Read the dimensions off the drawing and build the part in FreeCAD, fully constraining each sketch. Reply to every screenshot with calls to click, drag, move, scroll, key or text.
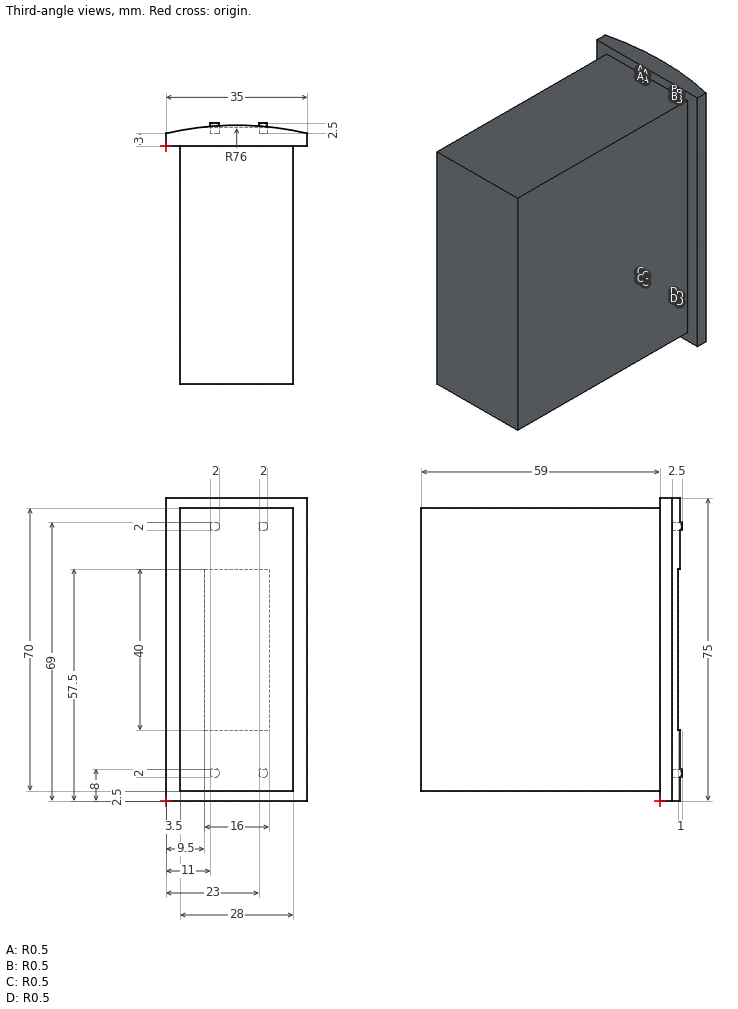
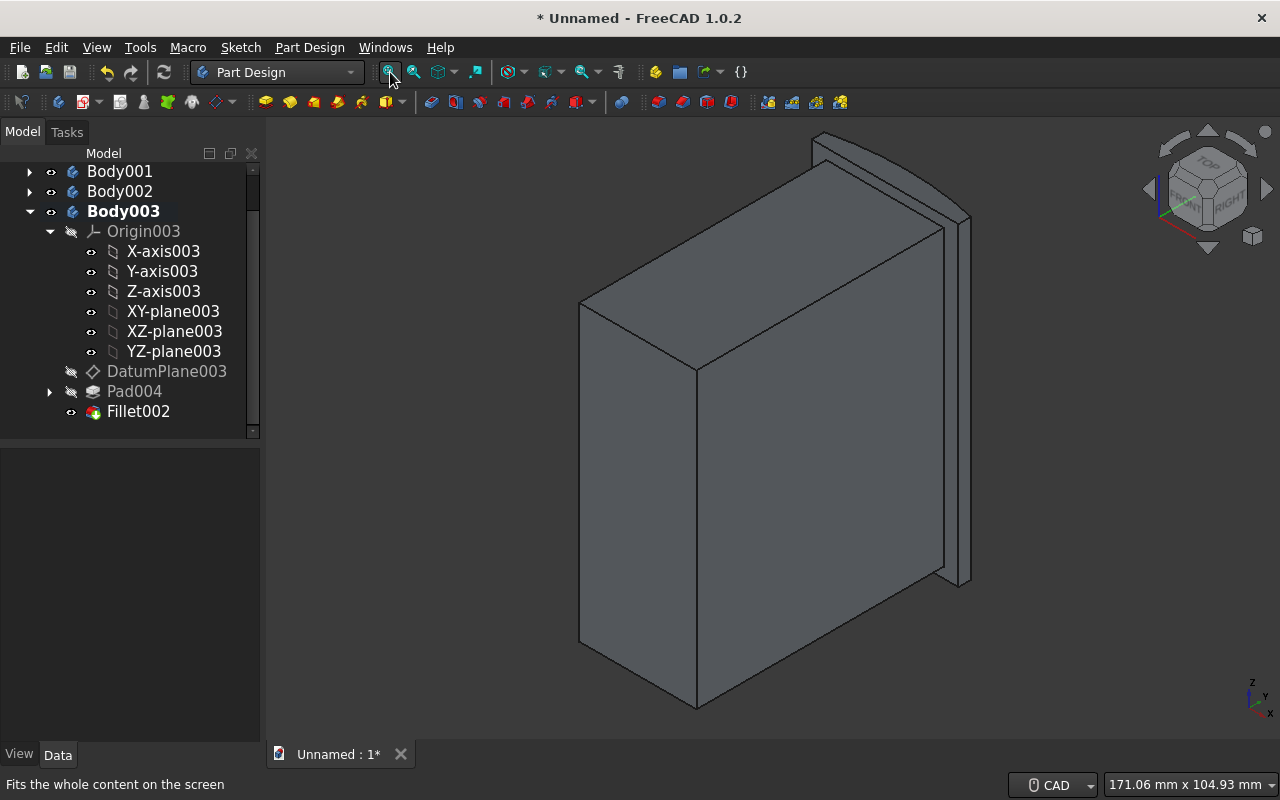
click(60, 102)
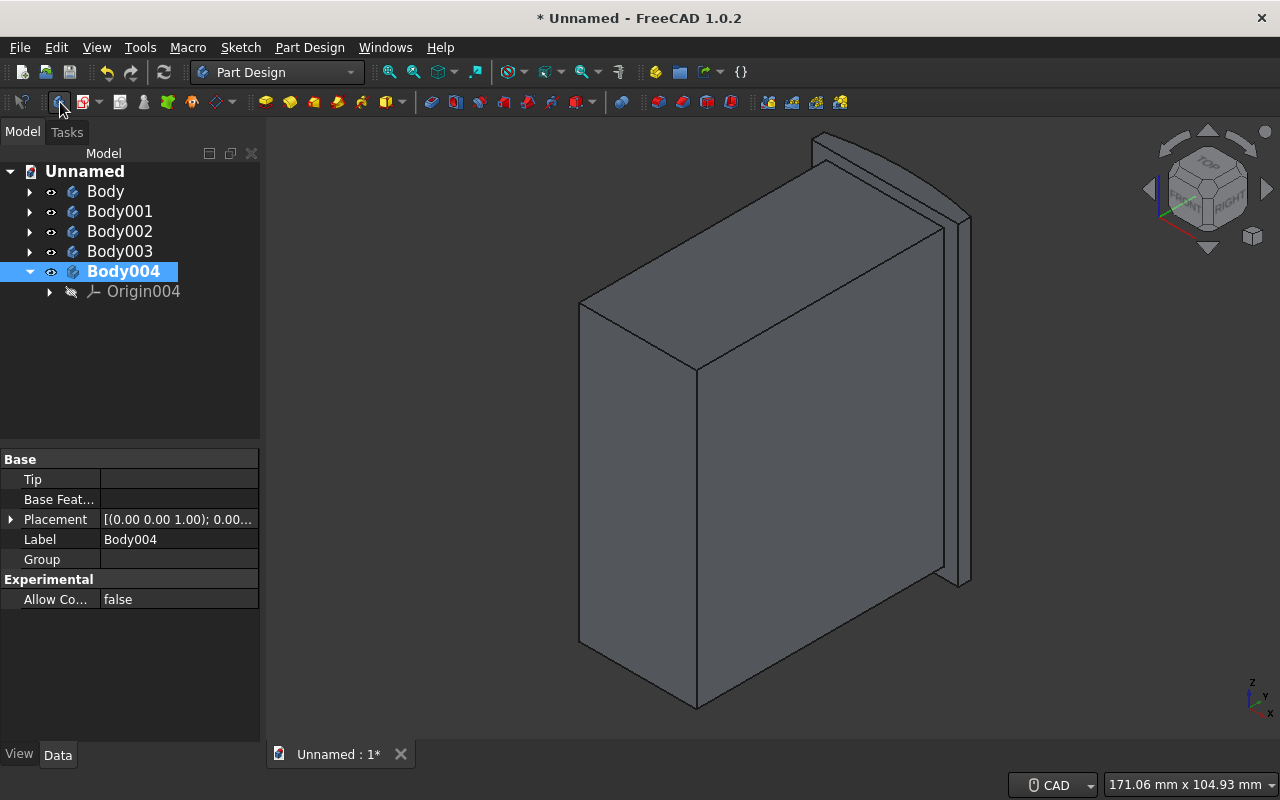
click(50, 292)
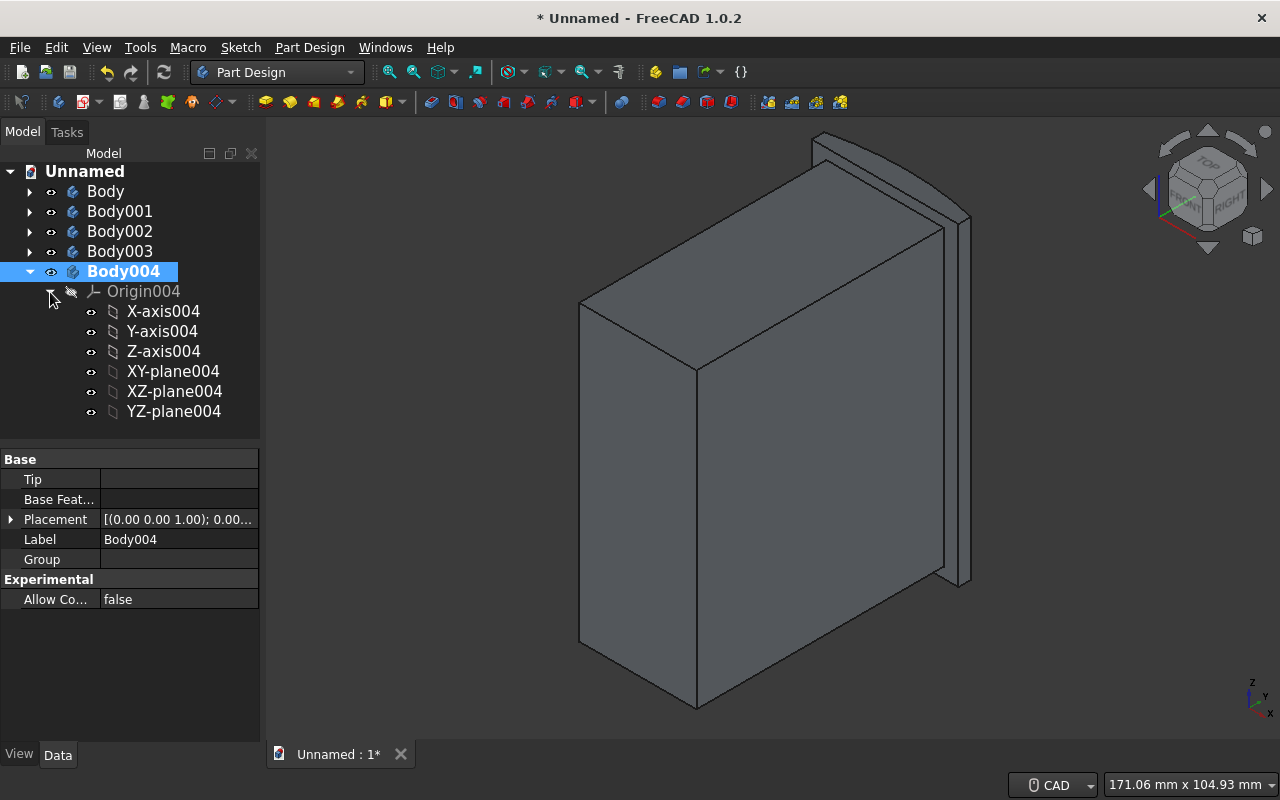
click(136, 392)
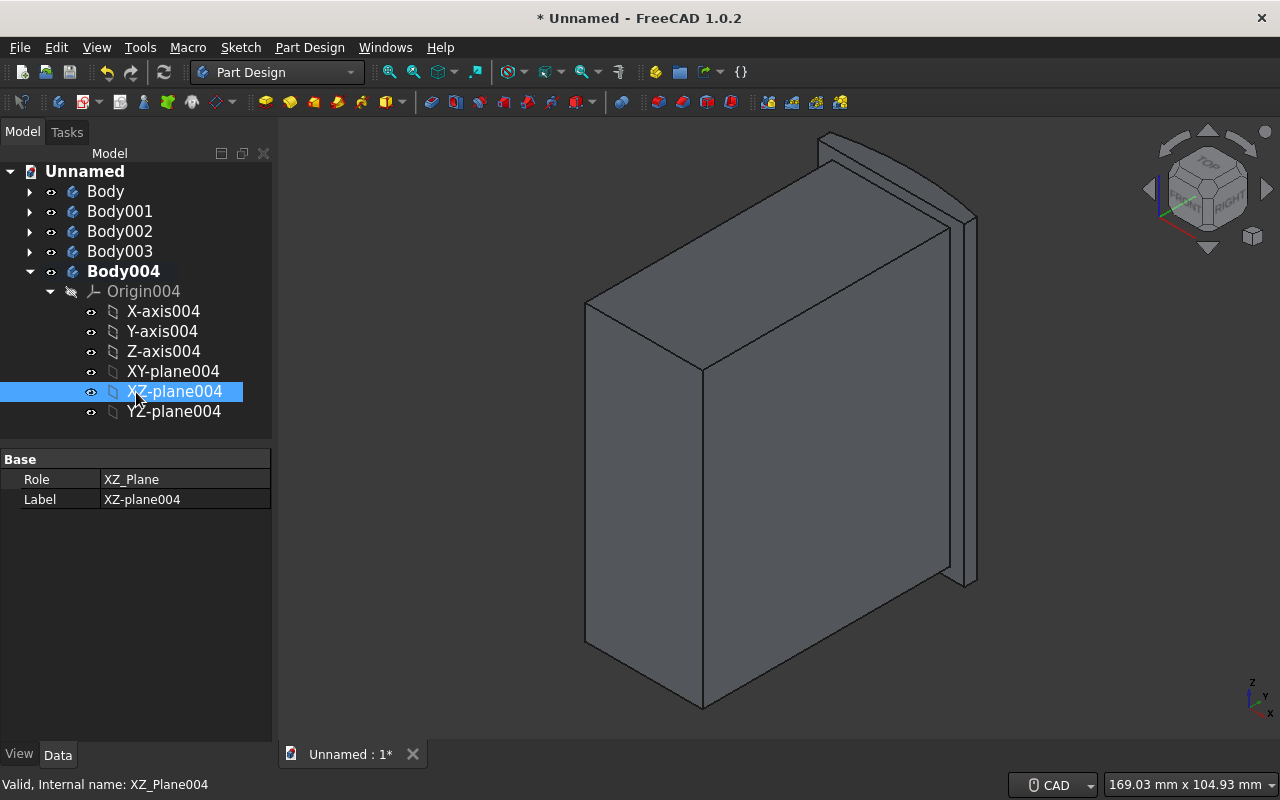
click(216, 102)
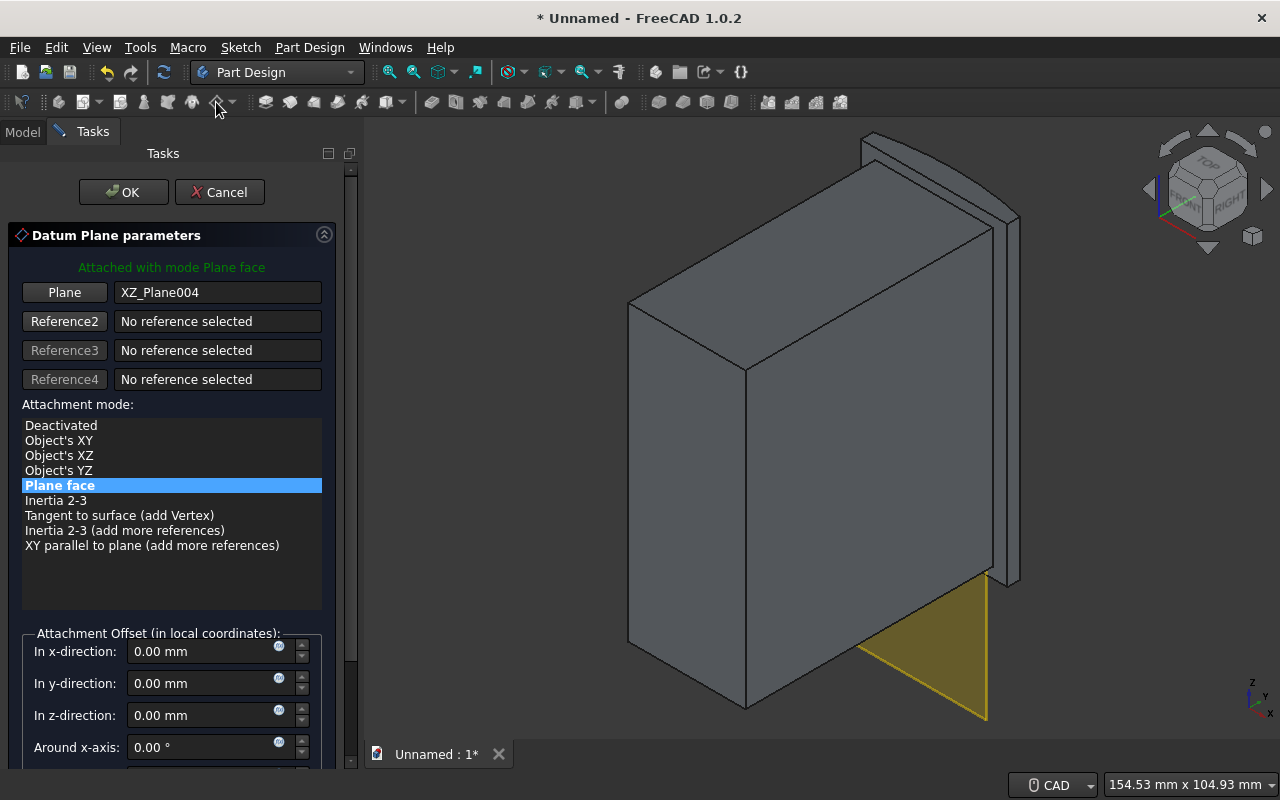
triple_click(210, 715)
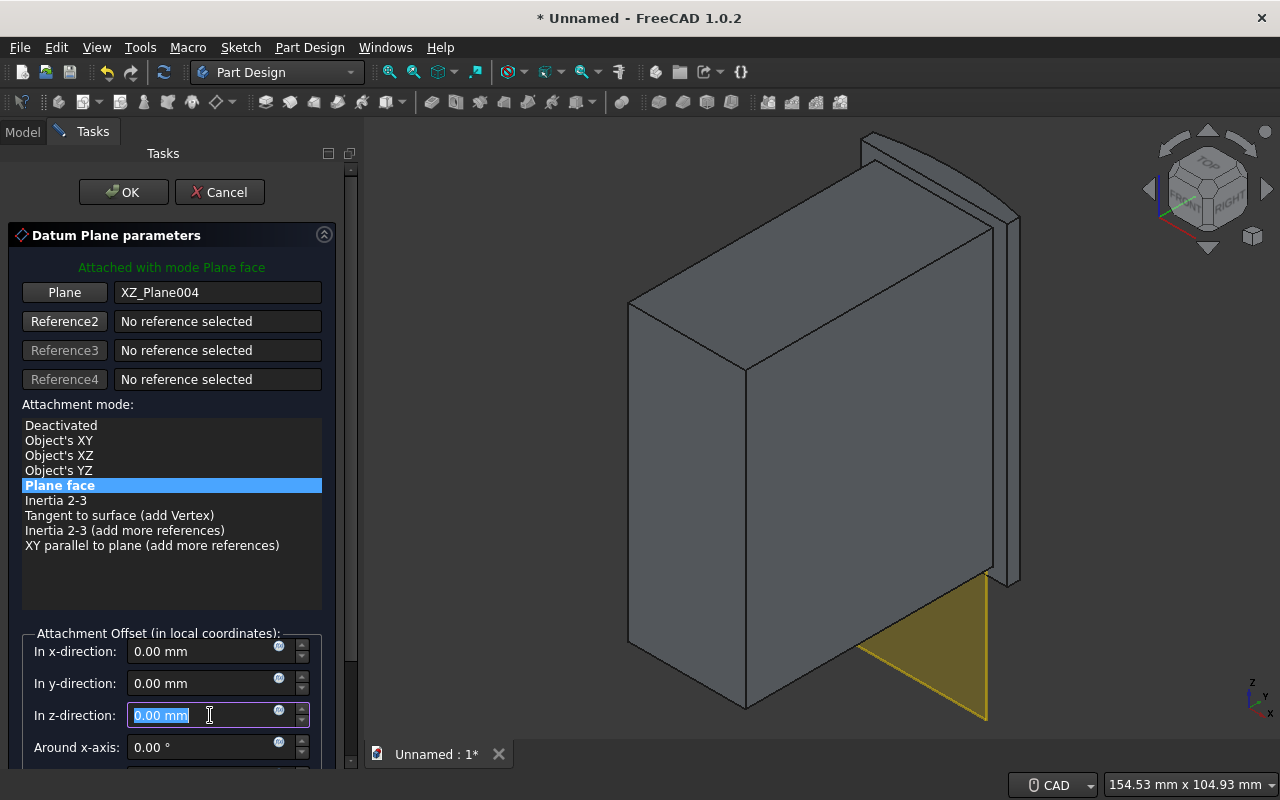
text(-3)
key(Tab)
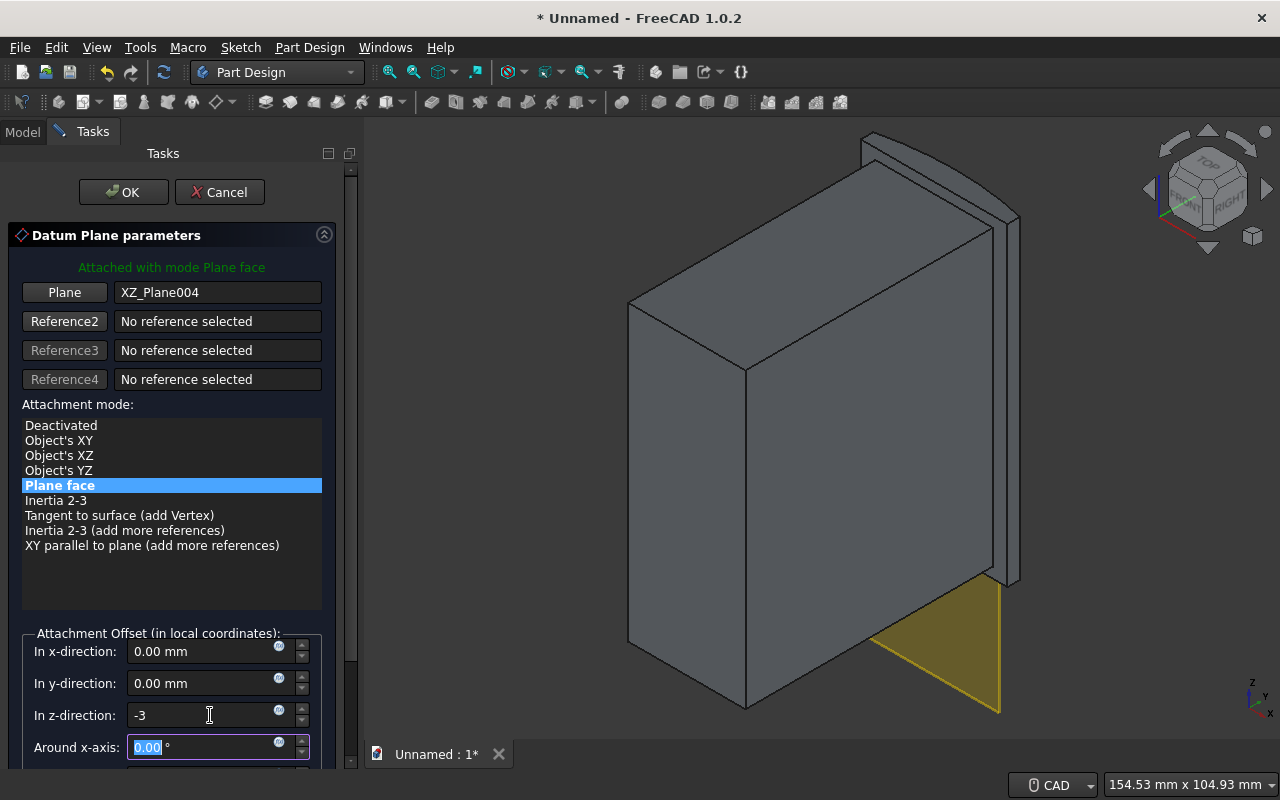
click(124, 192)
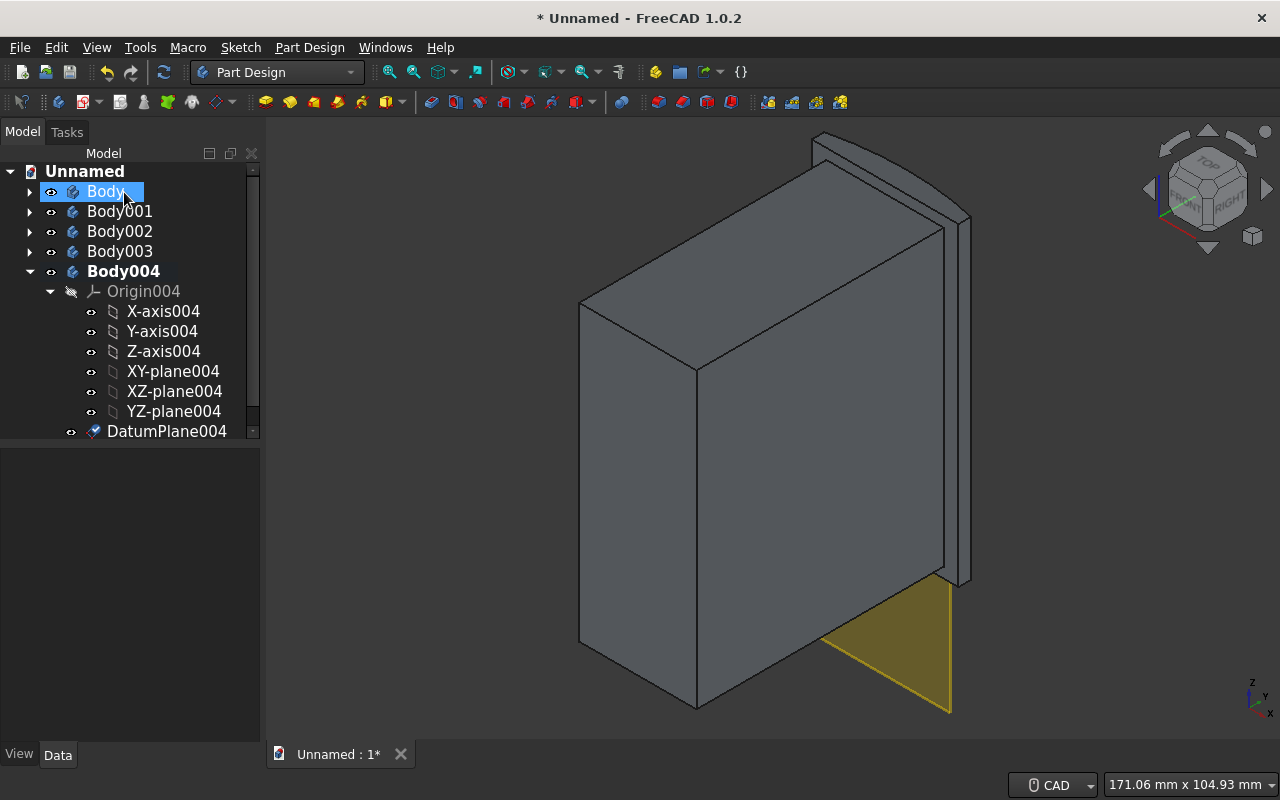
click(116, 432)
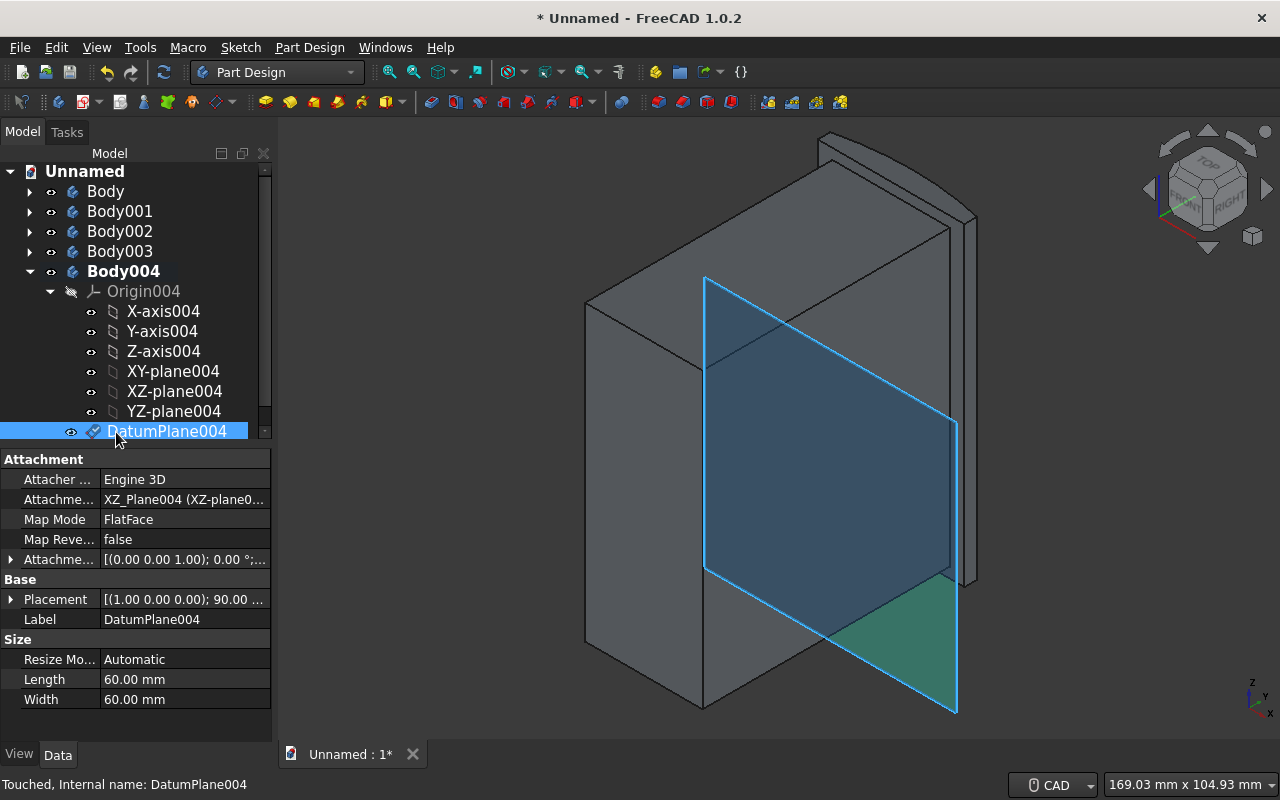
click(84, 102)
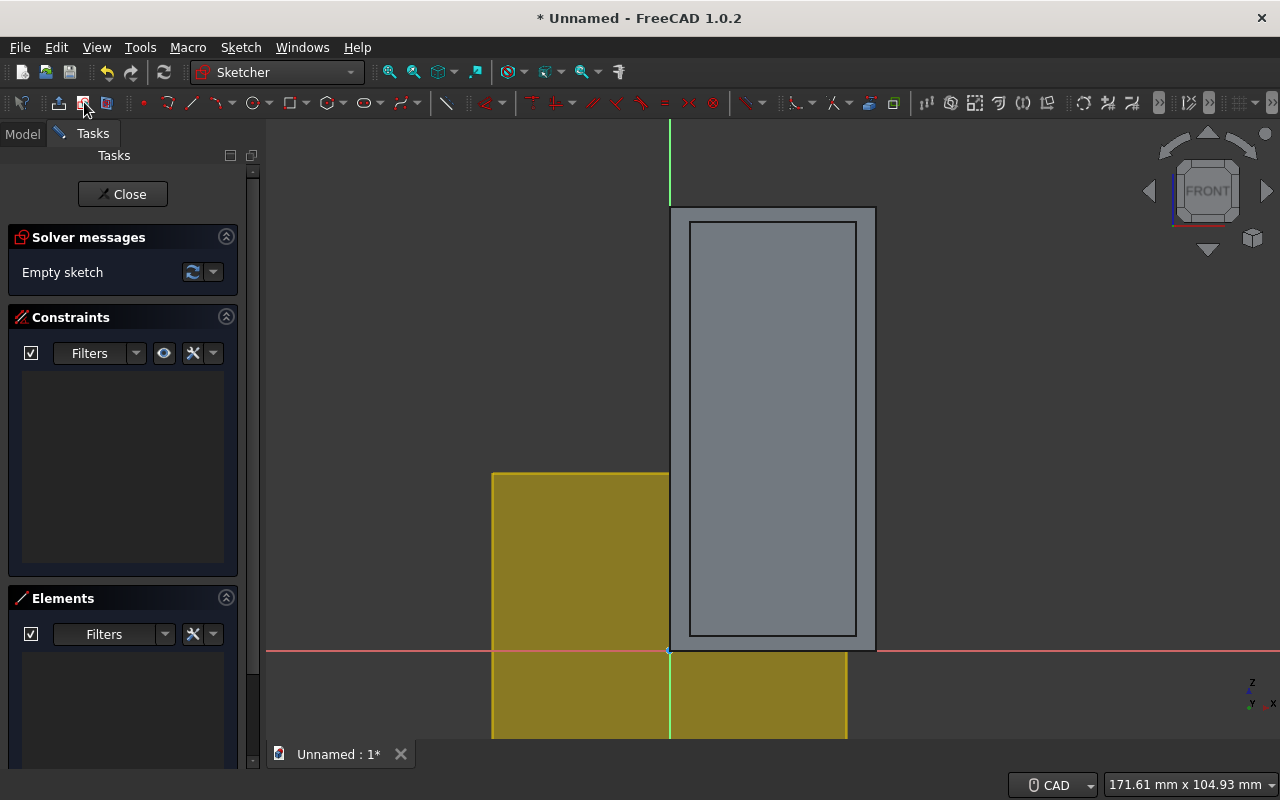
scroll(817, 619, up, 15)